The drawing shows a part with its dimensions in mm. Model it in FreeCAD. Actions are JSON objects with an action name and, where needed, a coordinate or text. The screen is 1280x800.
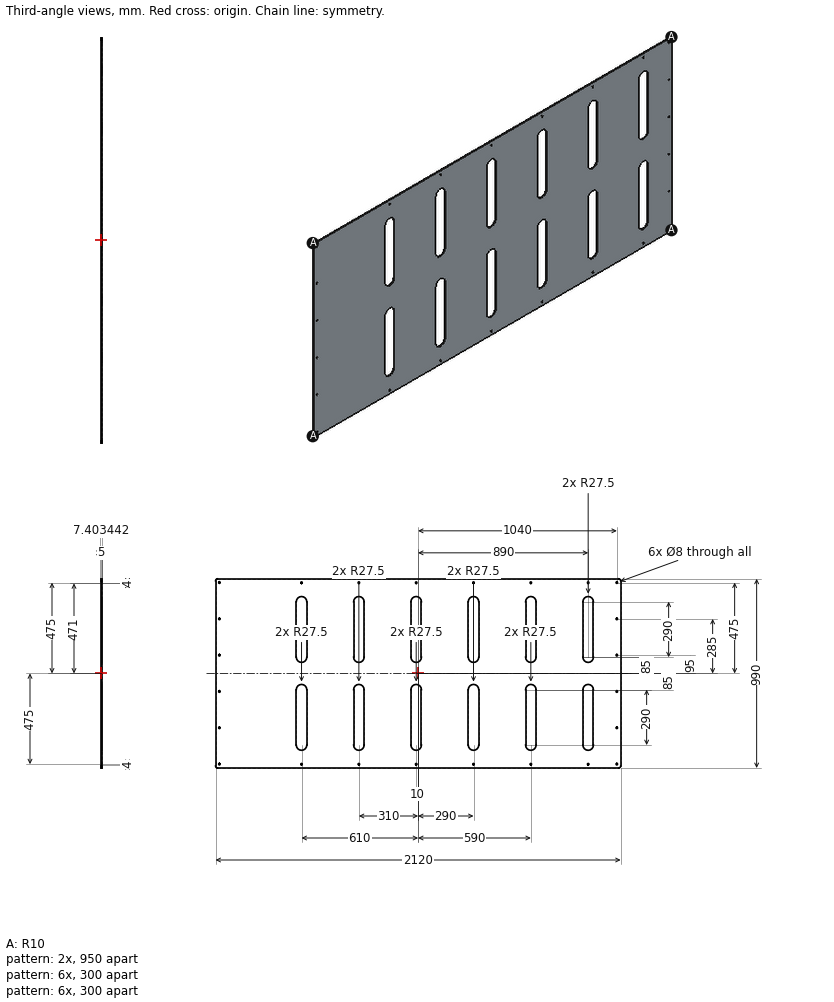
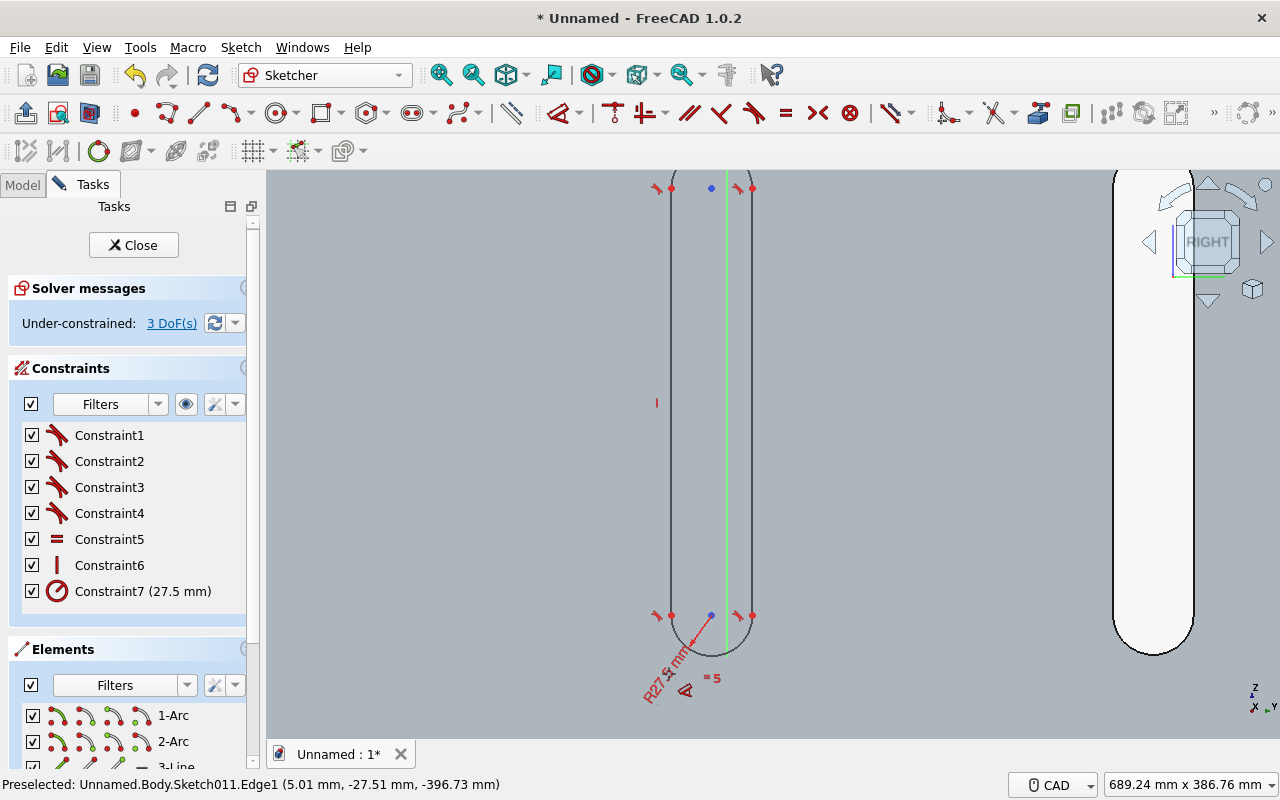
{"action": "left_click", "coordinate": [671, 487]}
{"action": "left_click", "coordinate": [637, 407]}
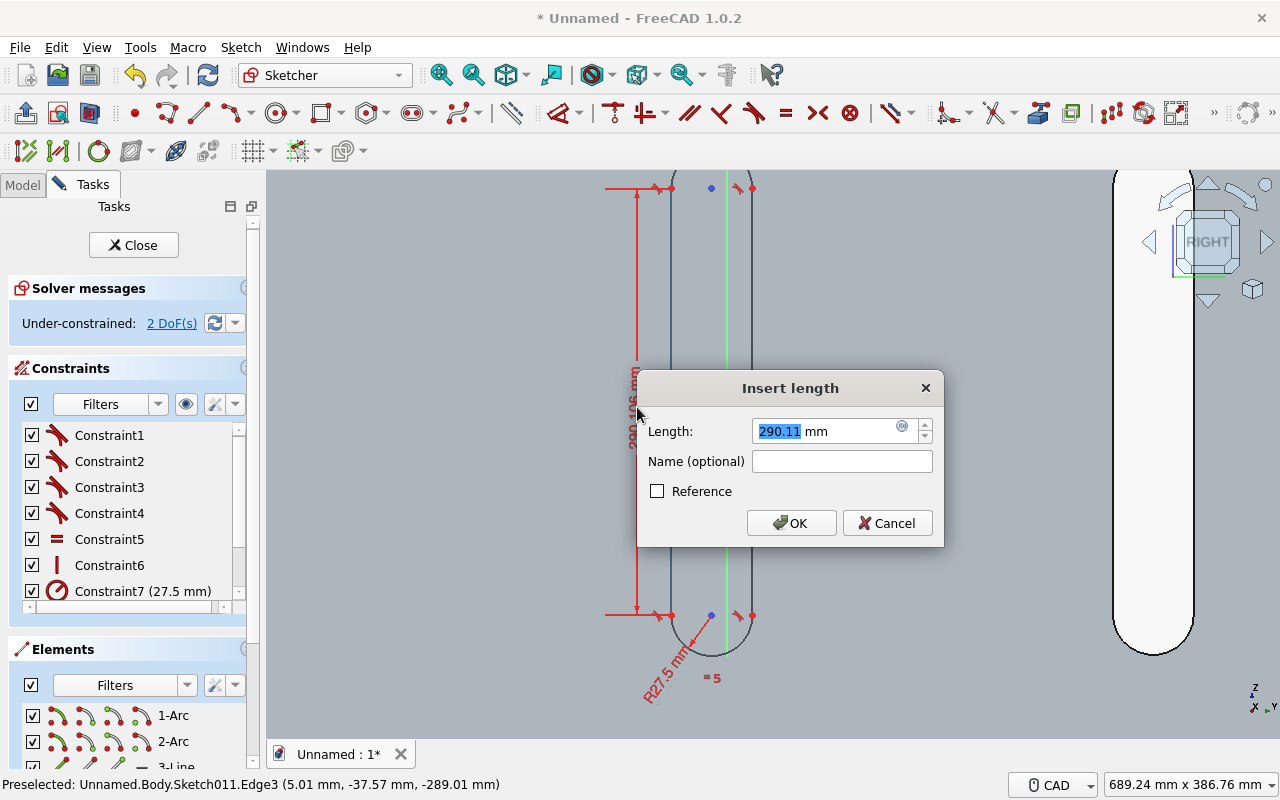
{"action": "type", "text": "290"}
{"action": "key", "text": "Return"}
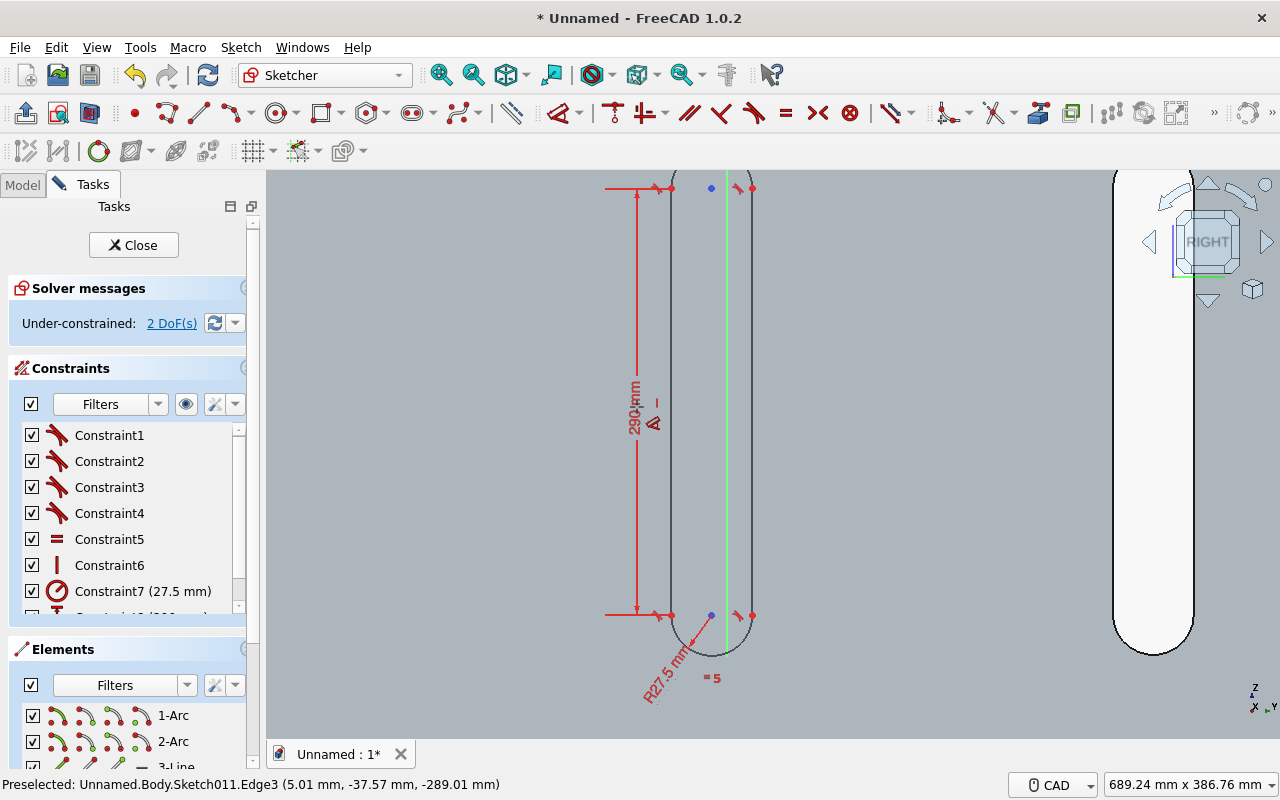
{"action": "scroll", "coordinate": [689, 649], "scroll_direction": "down", "scroll_amount": 2}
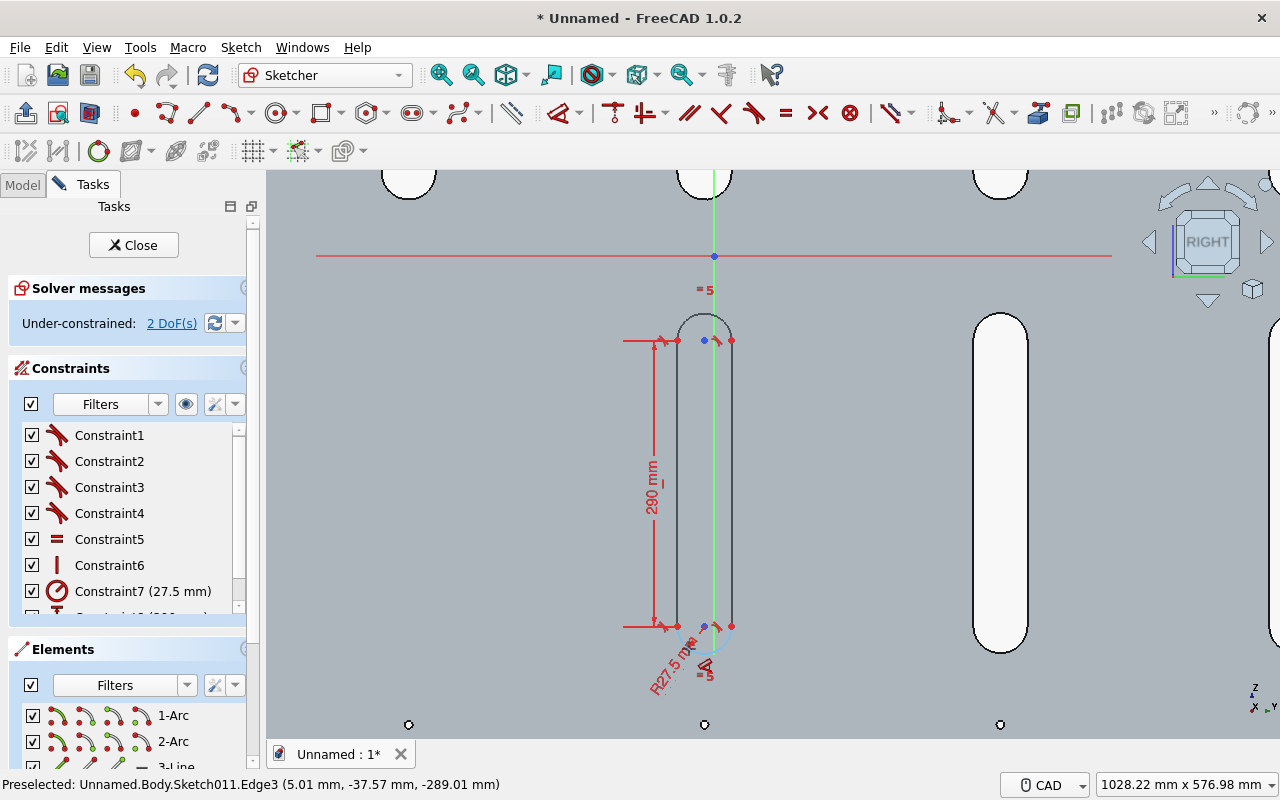
{"action": "left_click", "coordinate": [732, 341]}
{"action": "left_click", "coordinate": [766, 299]}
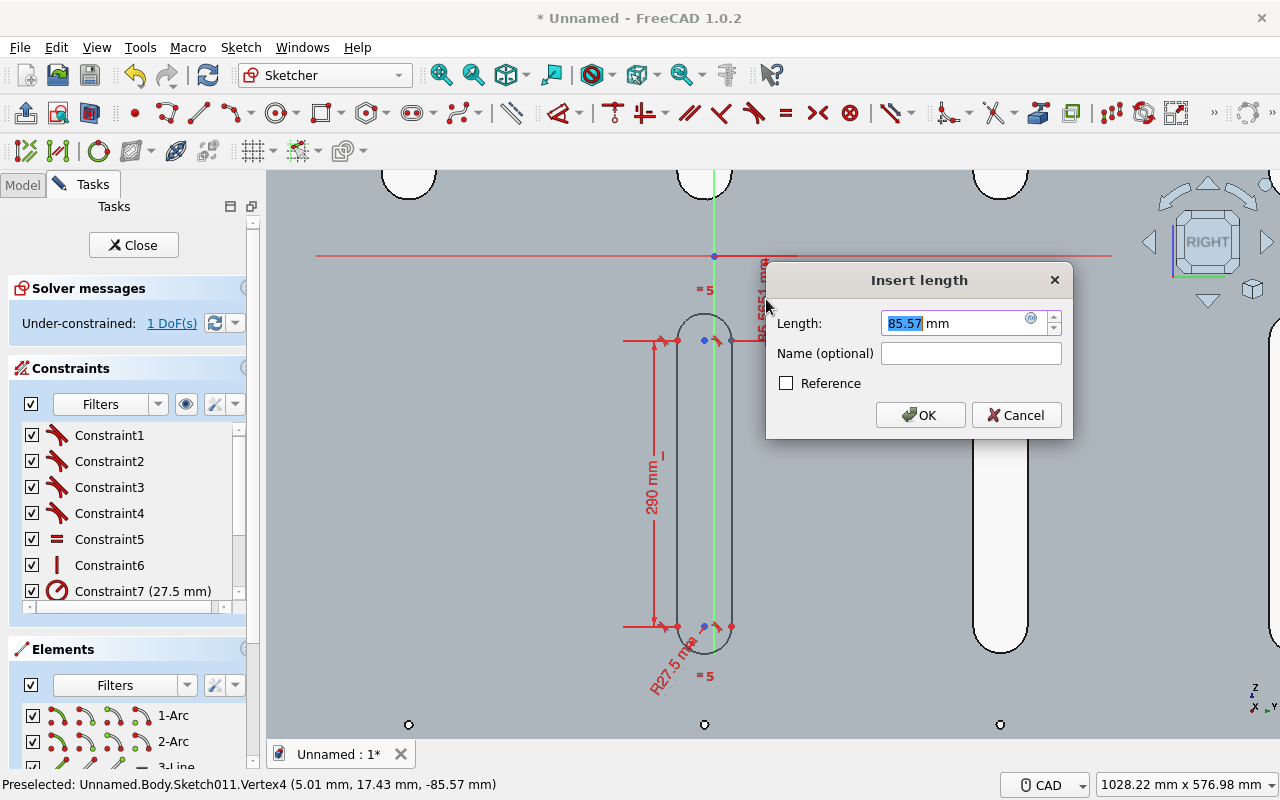
{"action": "type", "text": "85"}
{"action": "key", "text": "Return"}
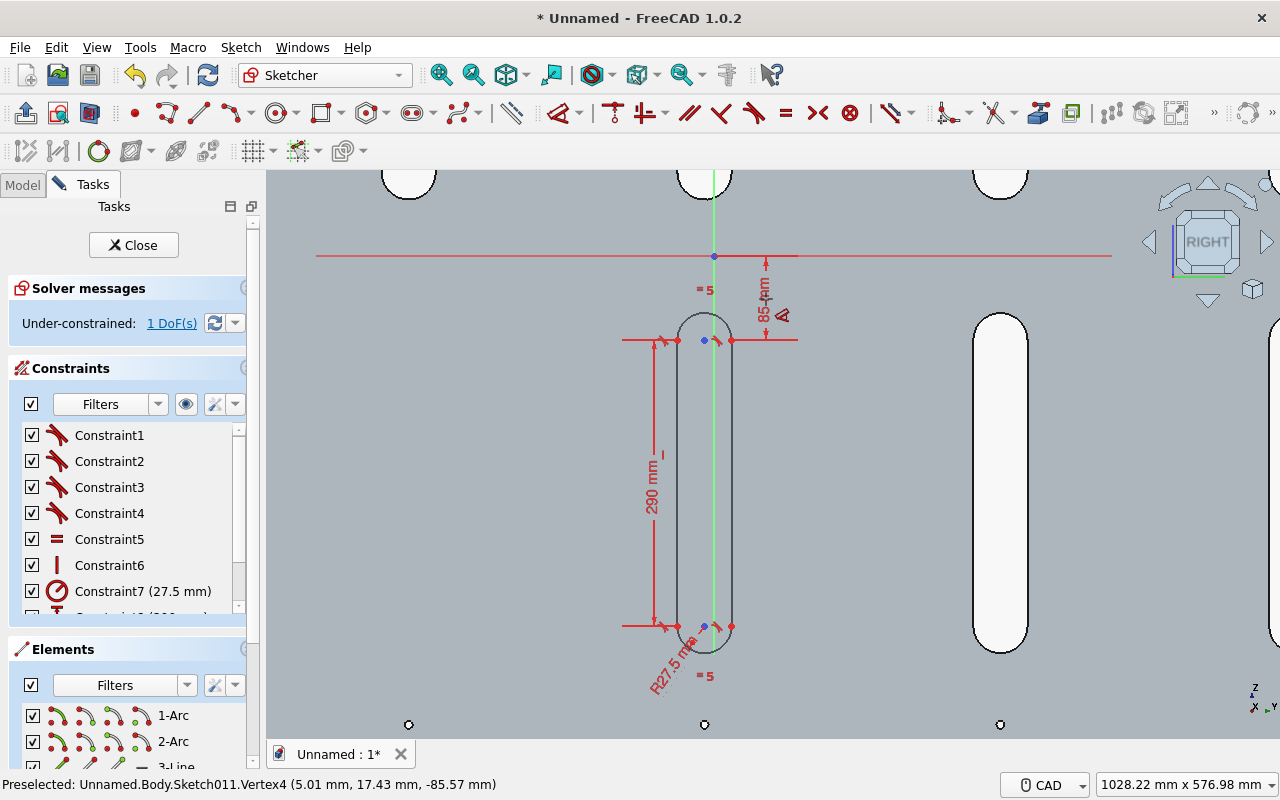
{"action": "scroll", "coordinate": [704, 626], "scroll_direction": "up", "scroll_amount": 7}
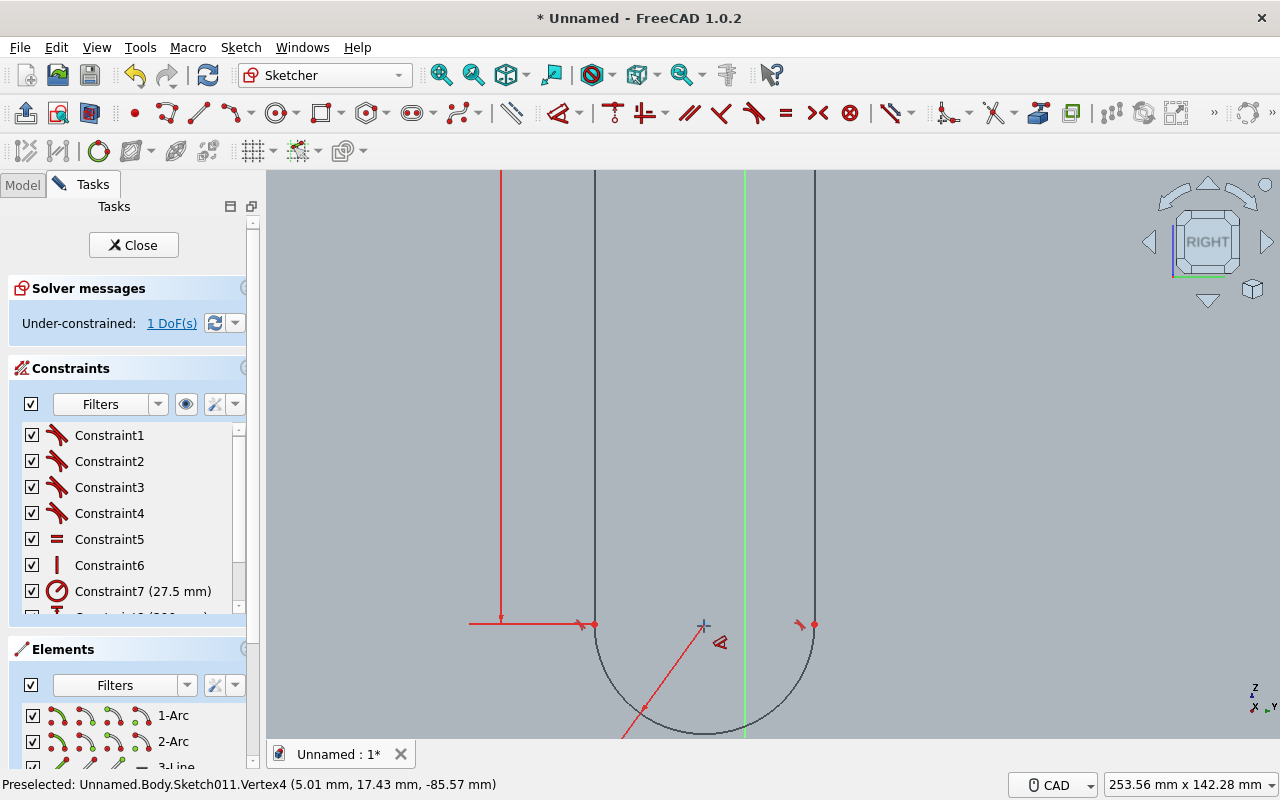
{"action": "left_click", "coordinate": [705, 624]}
{"action": "left_click", "coordinate": [725, 658]}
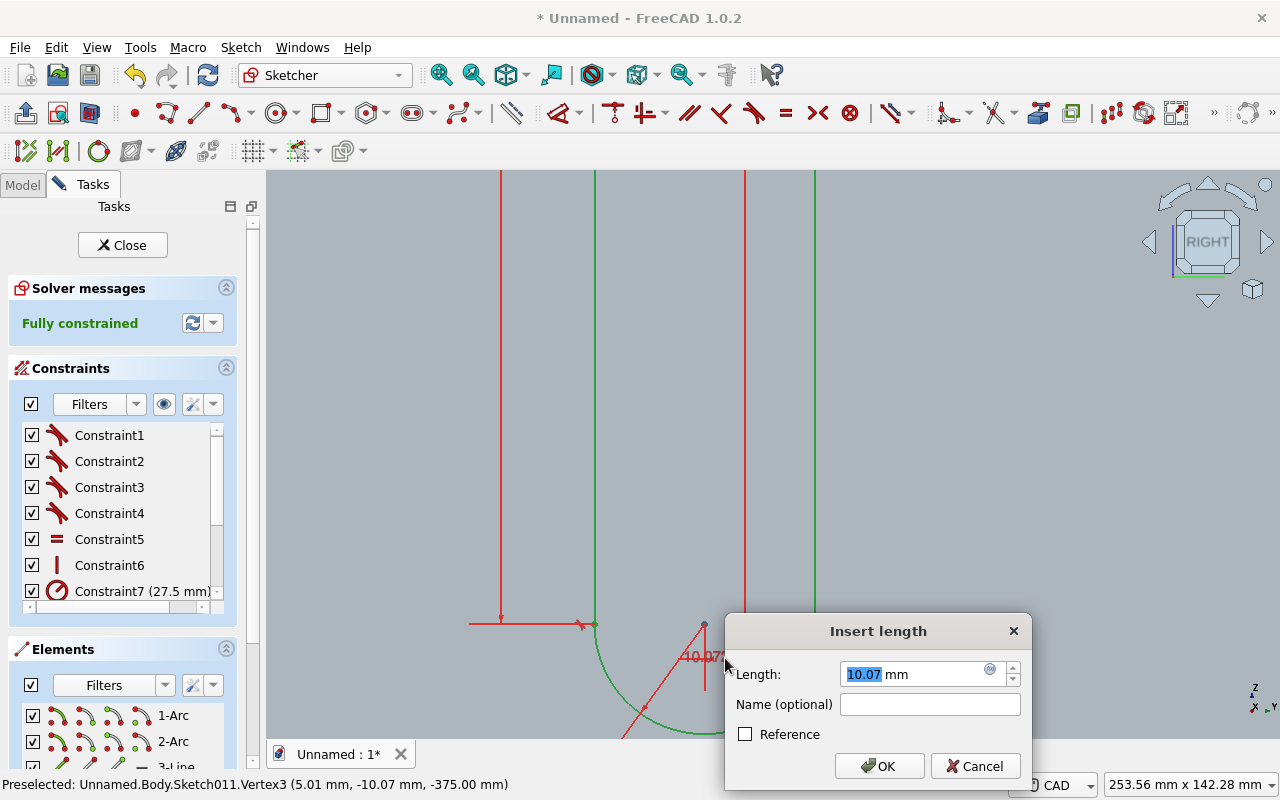
{"action": "type", "text": "10"}
{"action": "key", "text": "Return"}
{"action": "key", "text": "Escape"}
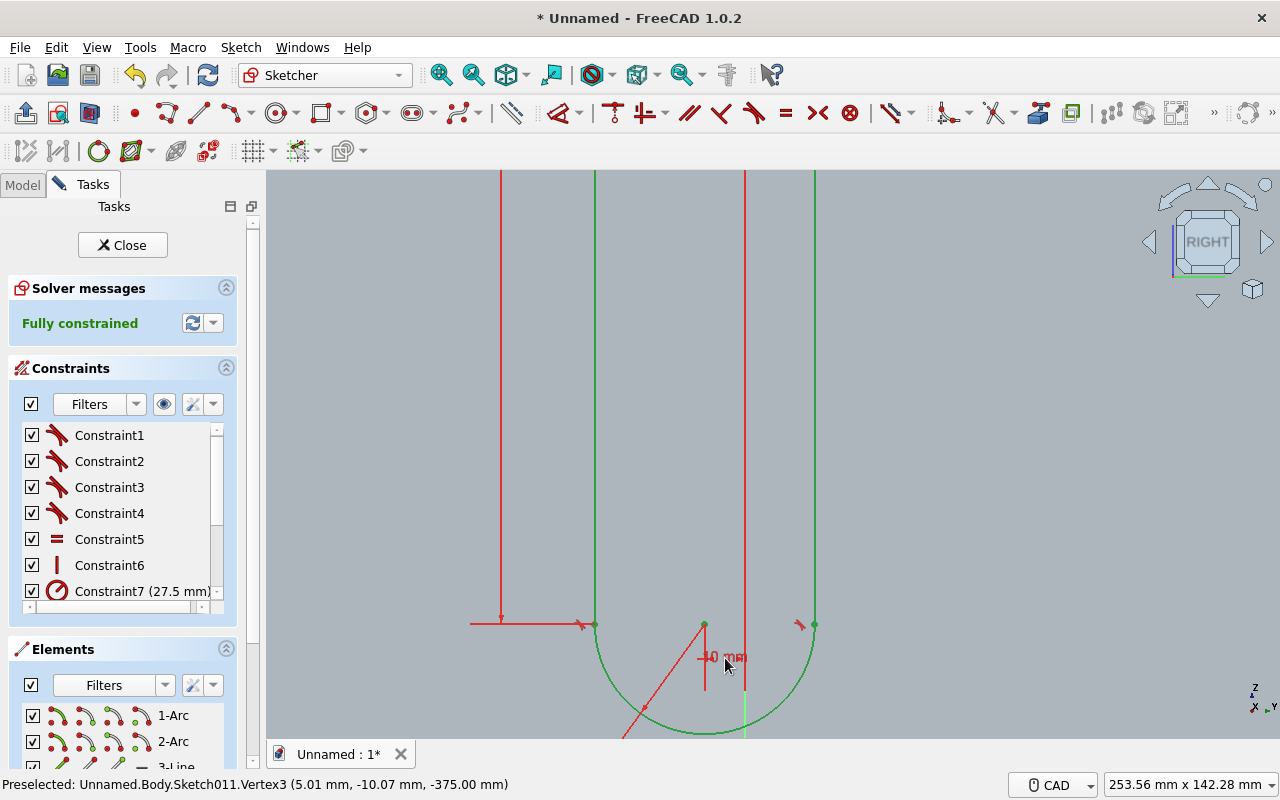
{"action": "left_click", "coordinate": [123, 245]}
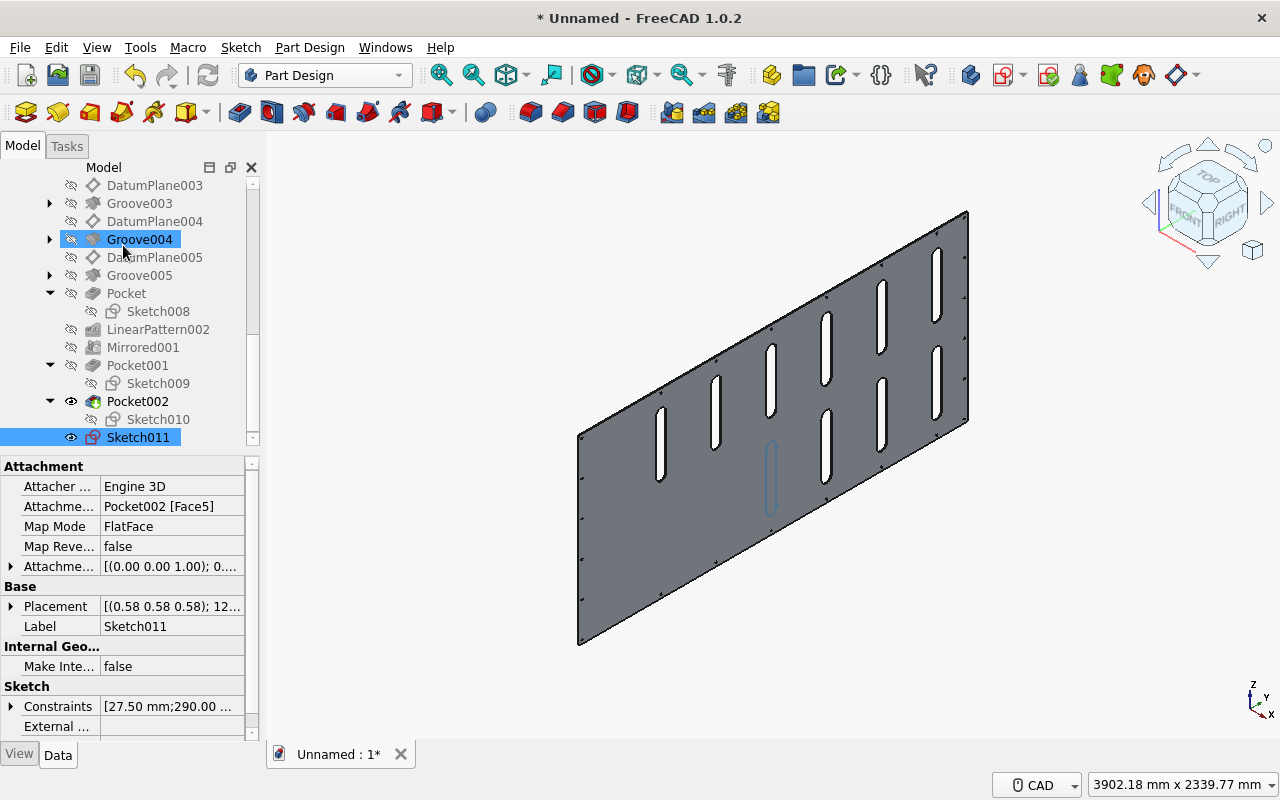
{"action": "left_click", "coordinate": [240, 112]}